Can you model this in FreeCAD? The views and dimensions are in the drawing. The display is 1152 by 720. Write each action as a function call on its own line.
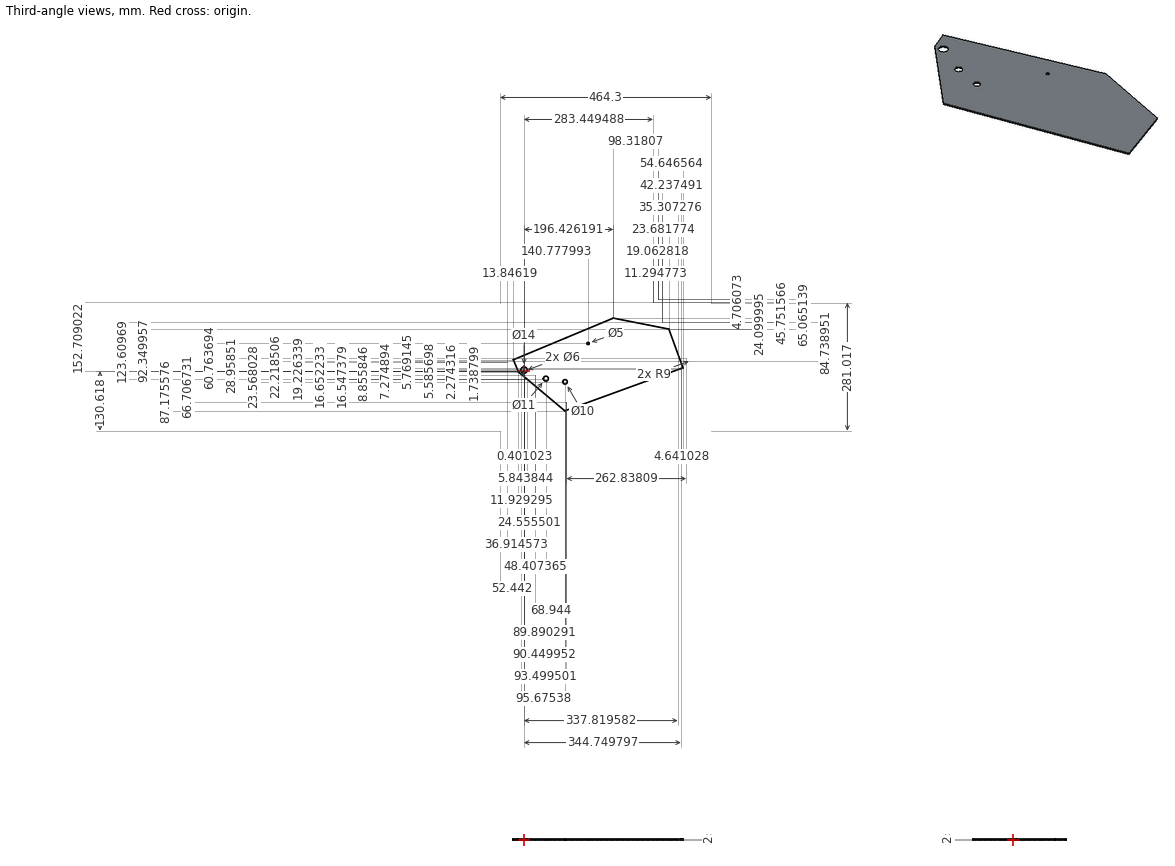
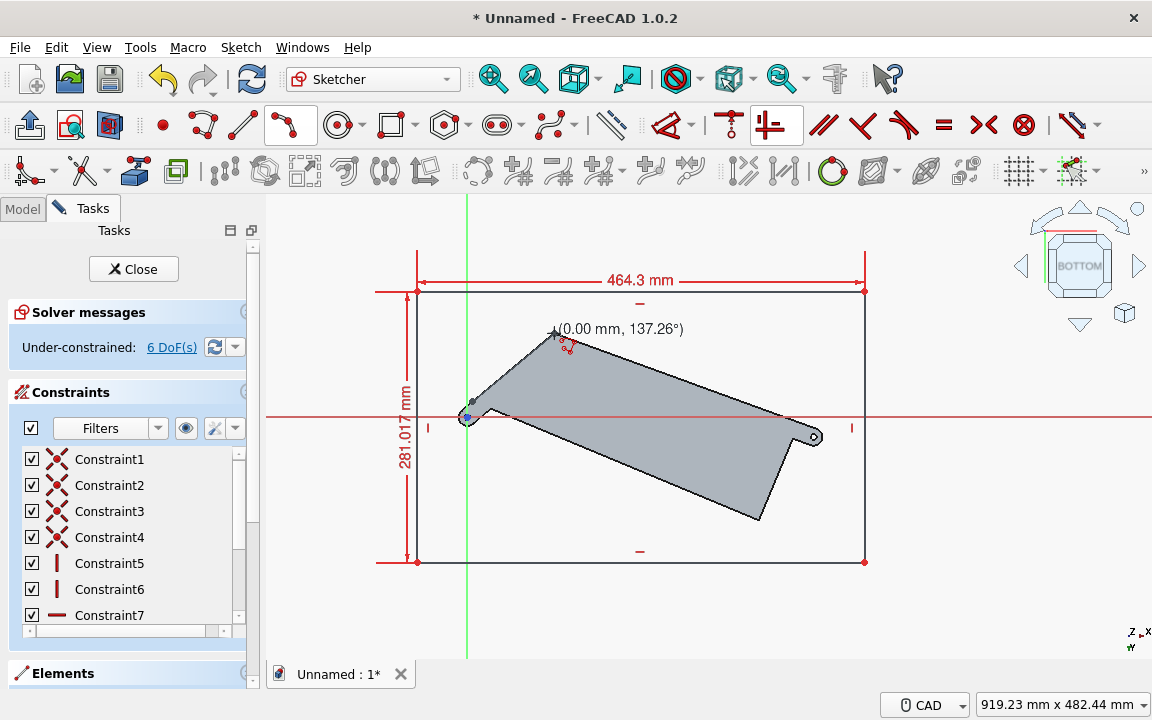
scroll(800, 423, up, 6)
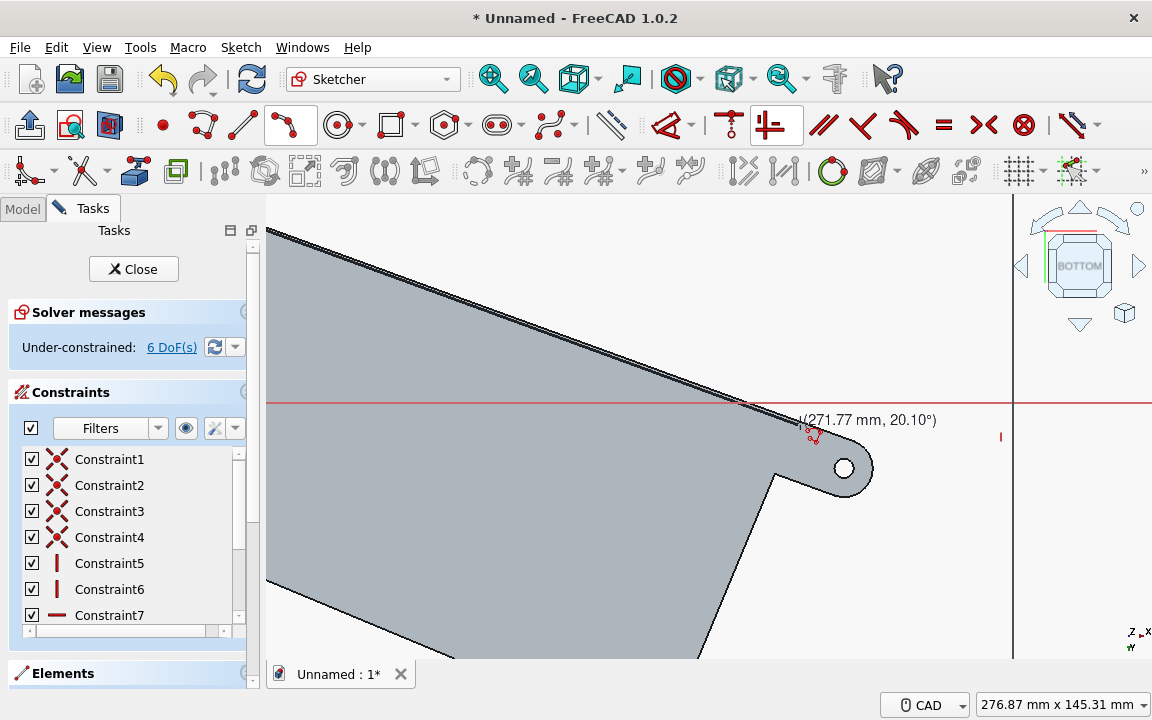
click(797, 421)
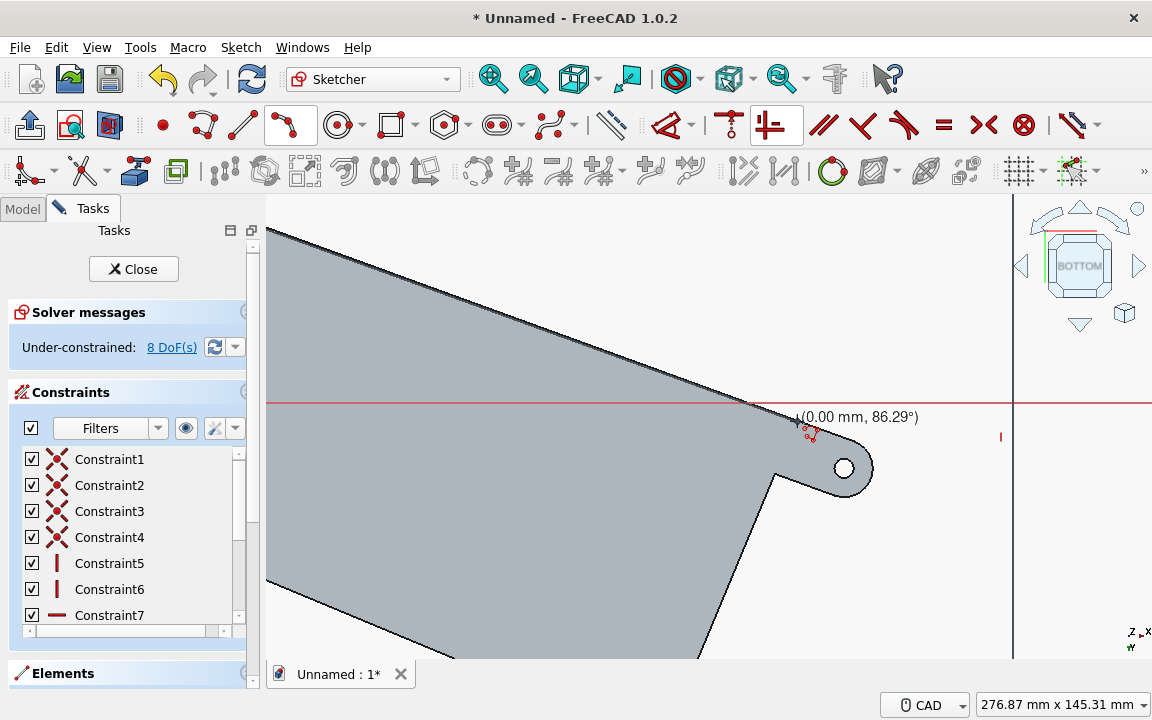
scroll(801, 423, down, 6)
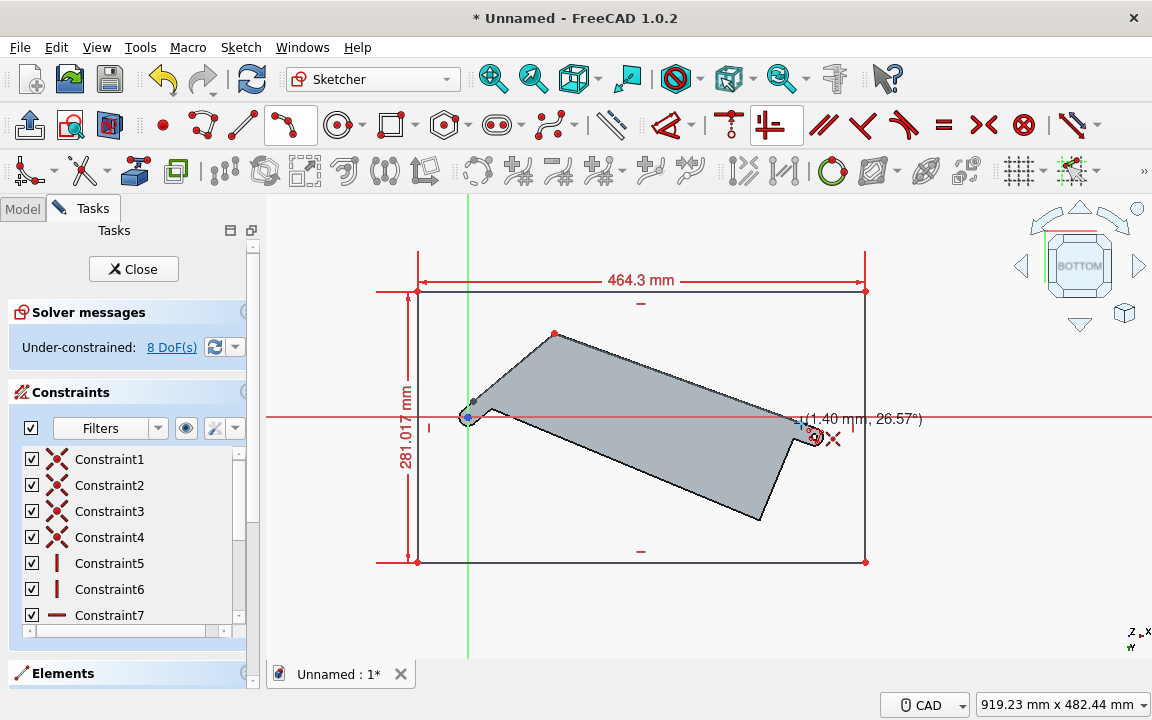
click(760, 520)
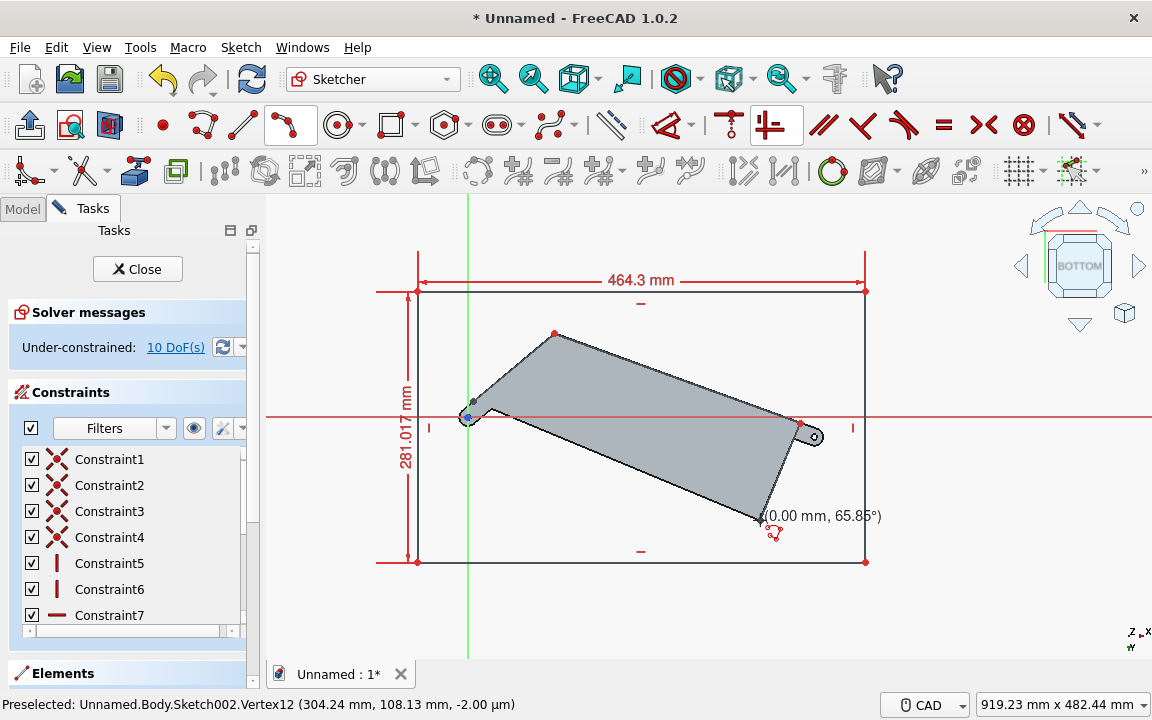
scroll(474, 401, up, 6)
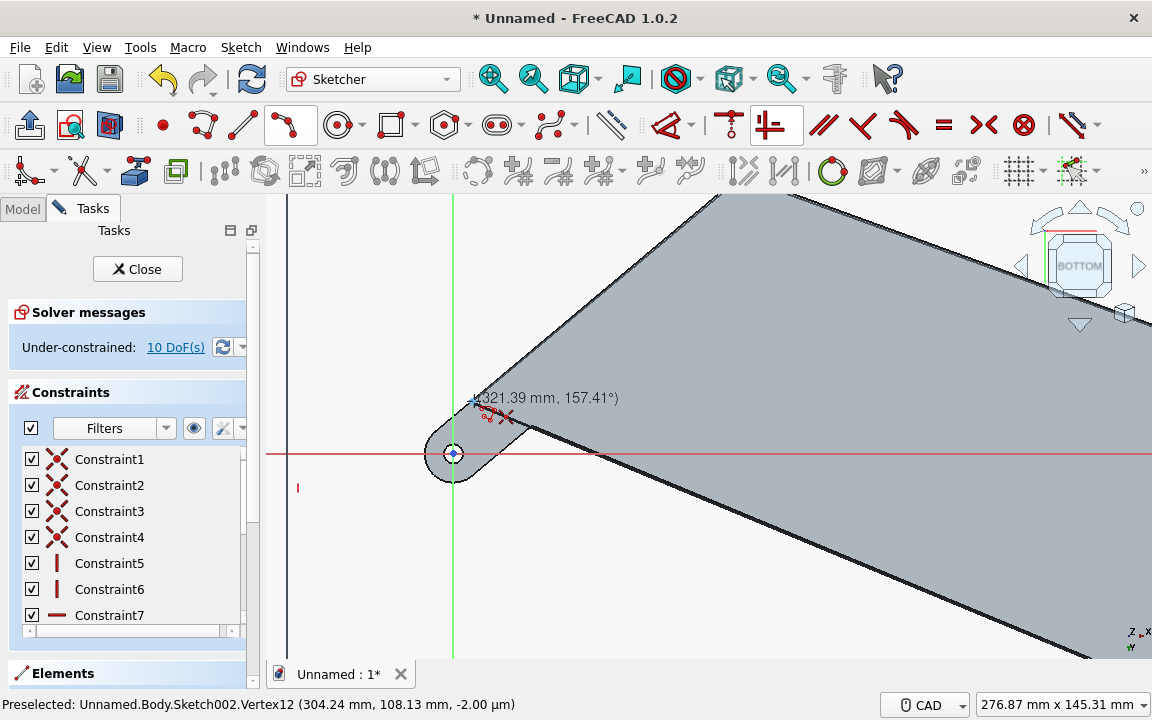
click(472, 402)
key(Escape)
key(Escape)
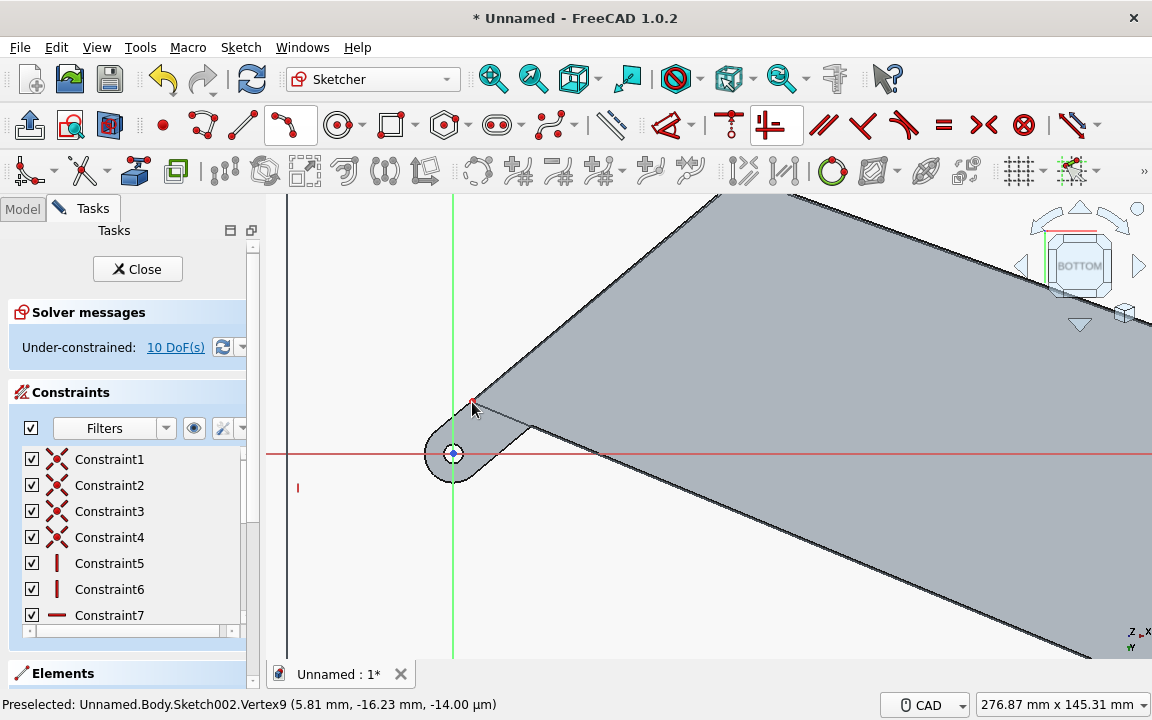
scroll(473, 401, down, 6)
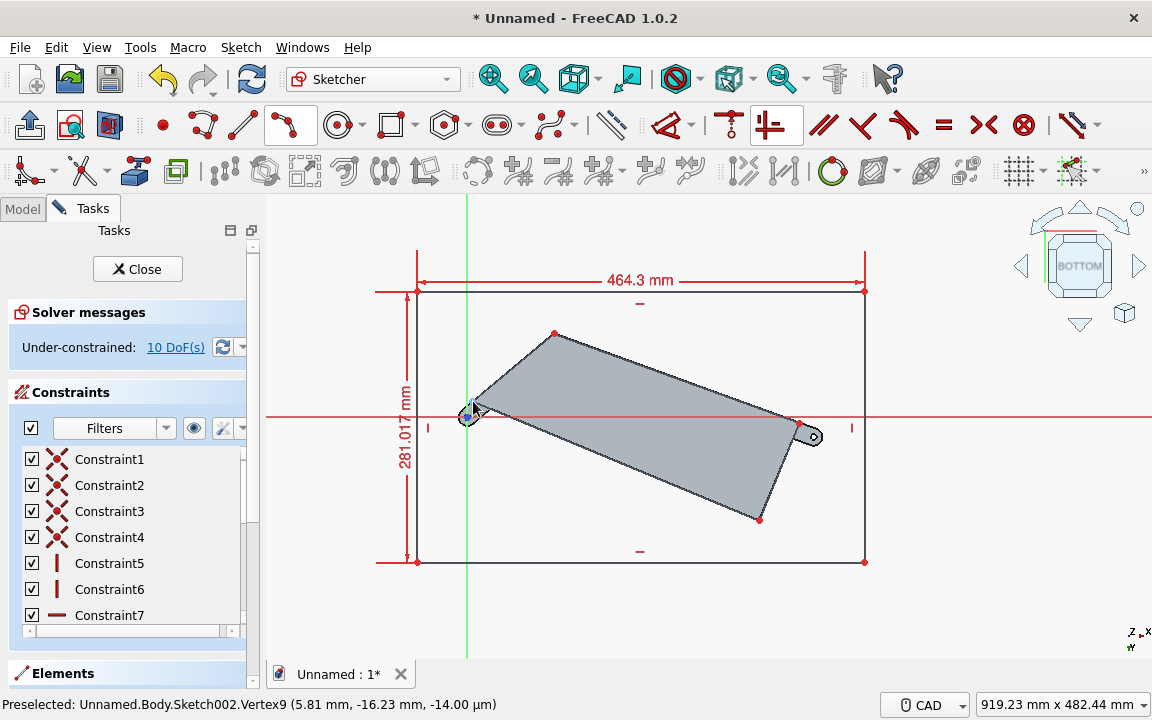
click(417, 292)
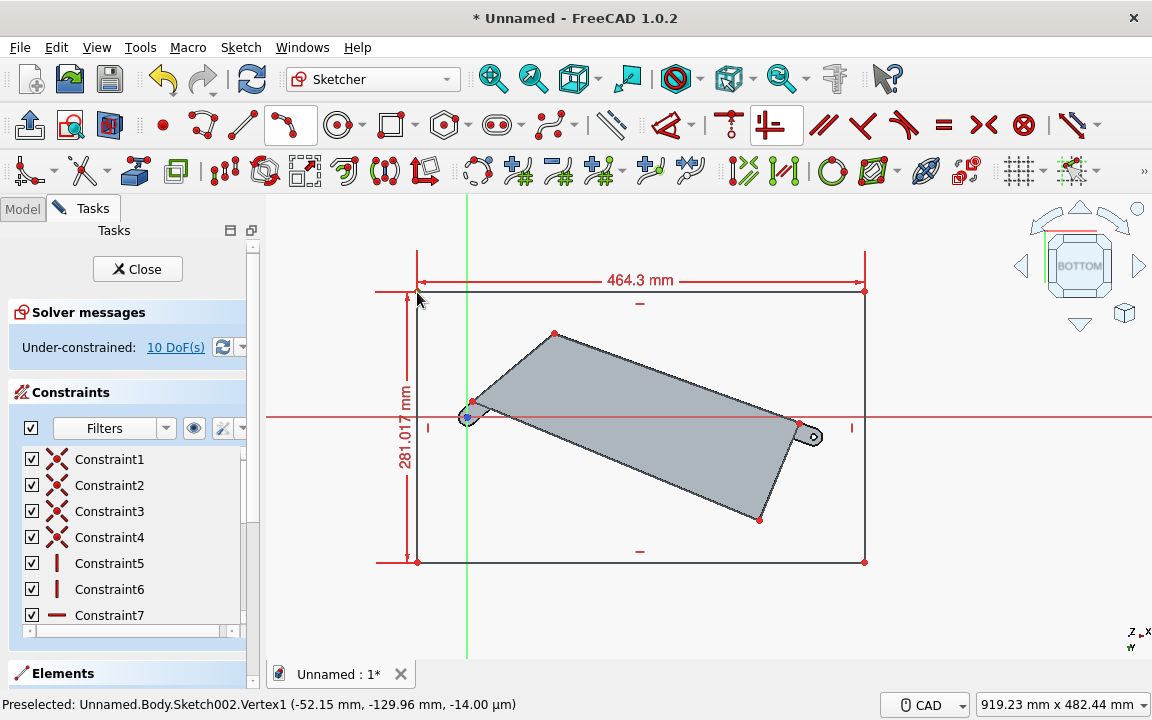
key(l)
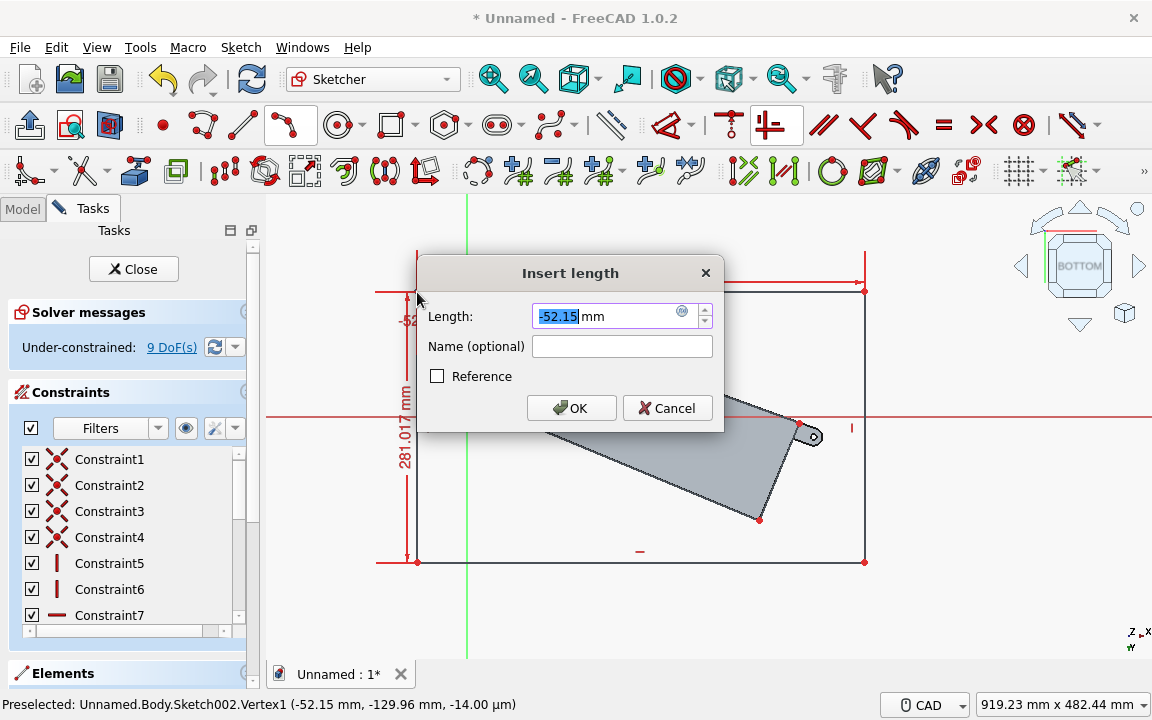
text(-52.442)
key(Return)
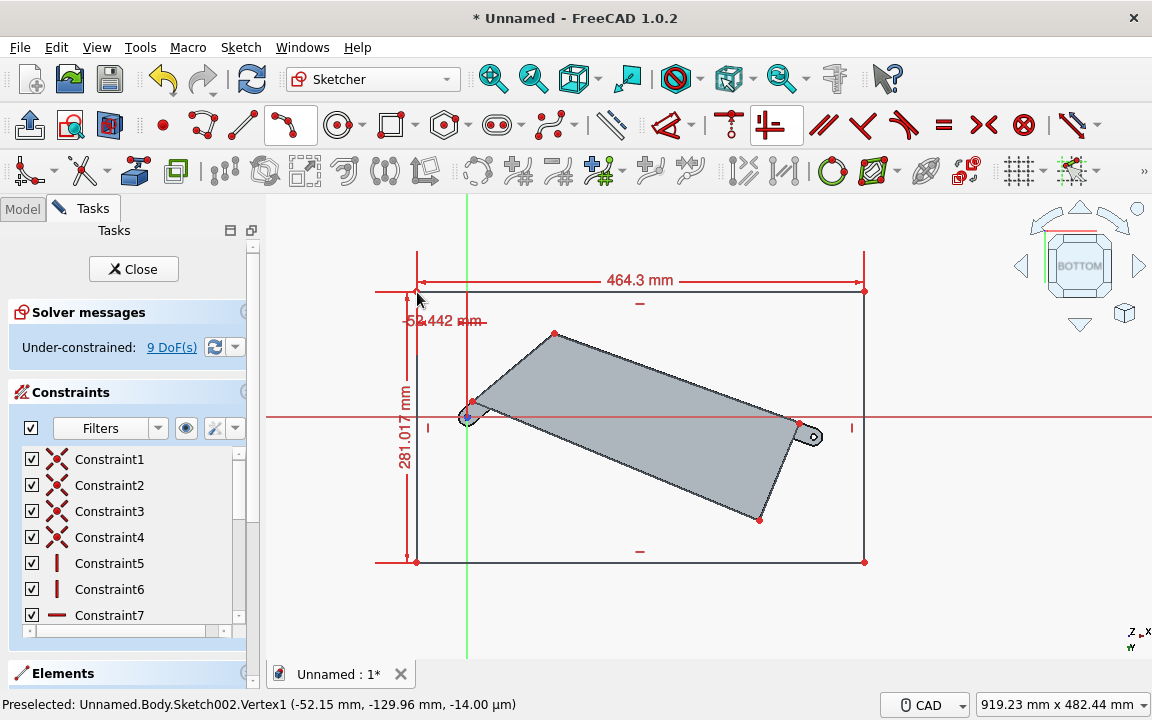
click(417, 292)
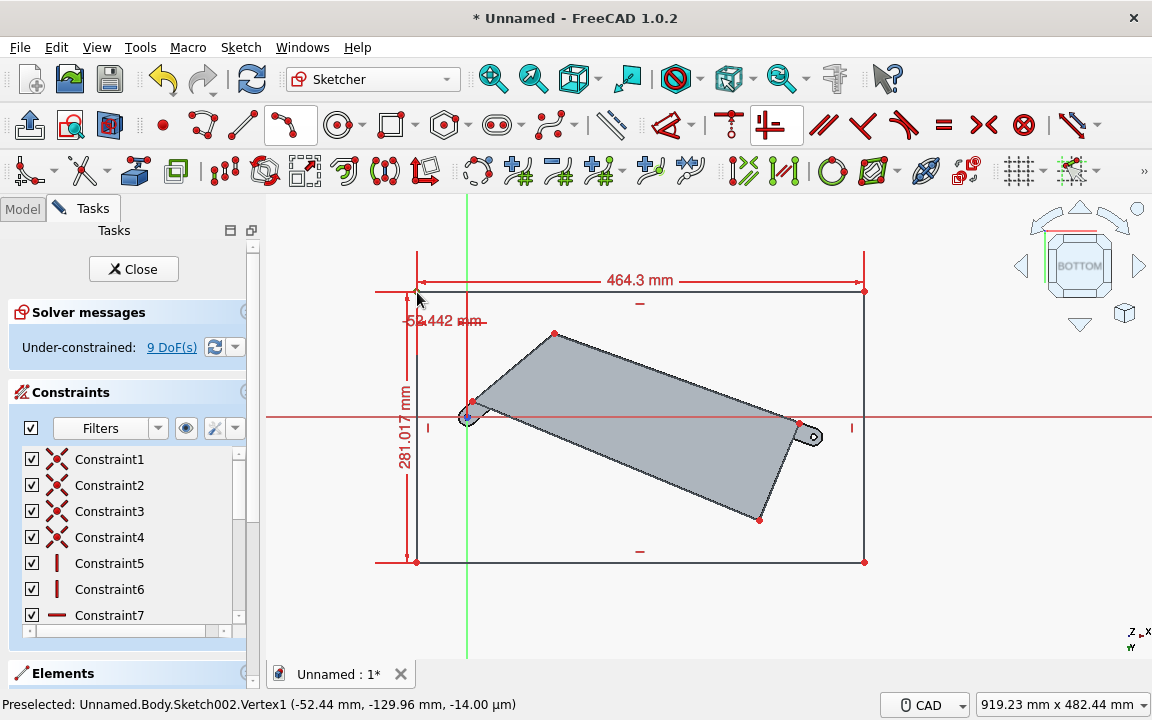
key(i)